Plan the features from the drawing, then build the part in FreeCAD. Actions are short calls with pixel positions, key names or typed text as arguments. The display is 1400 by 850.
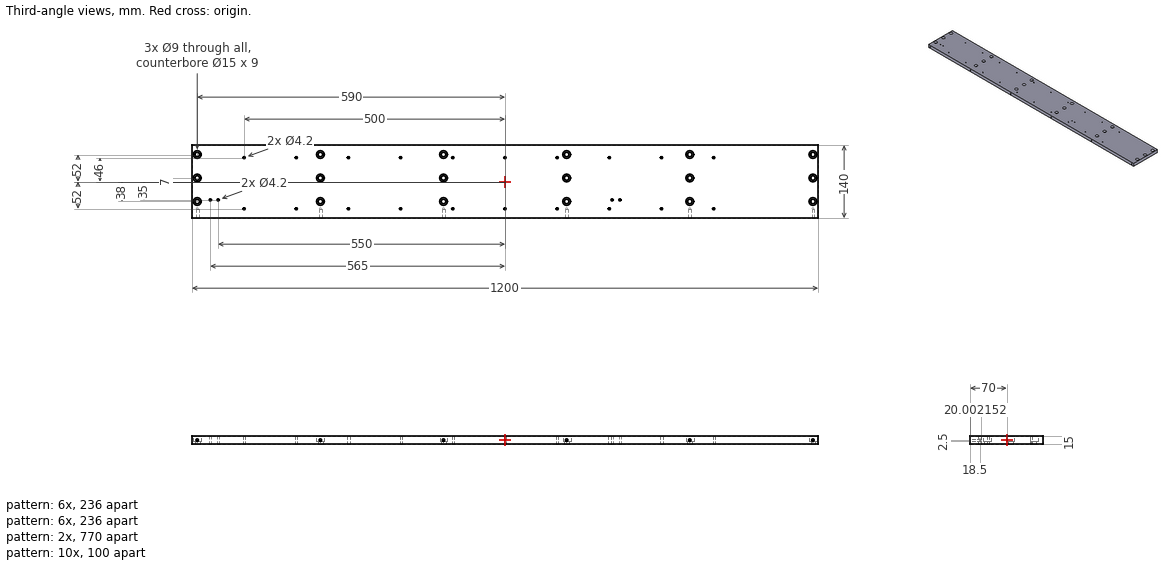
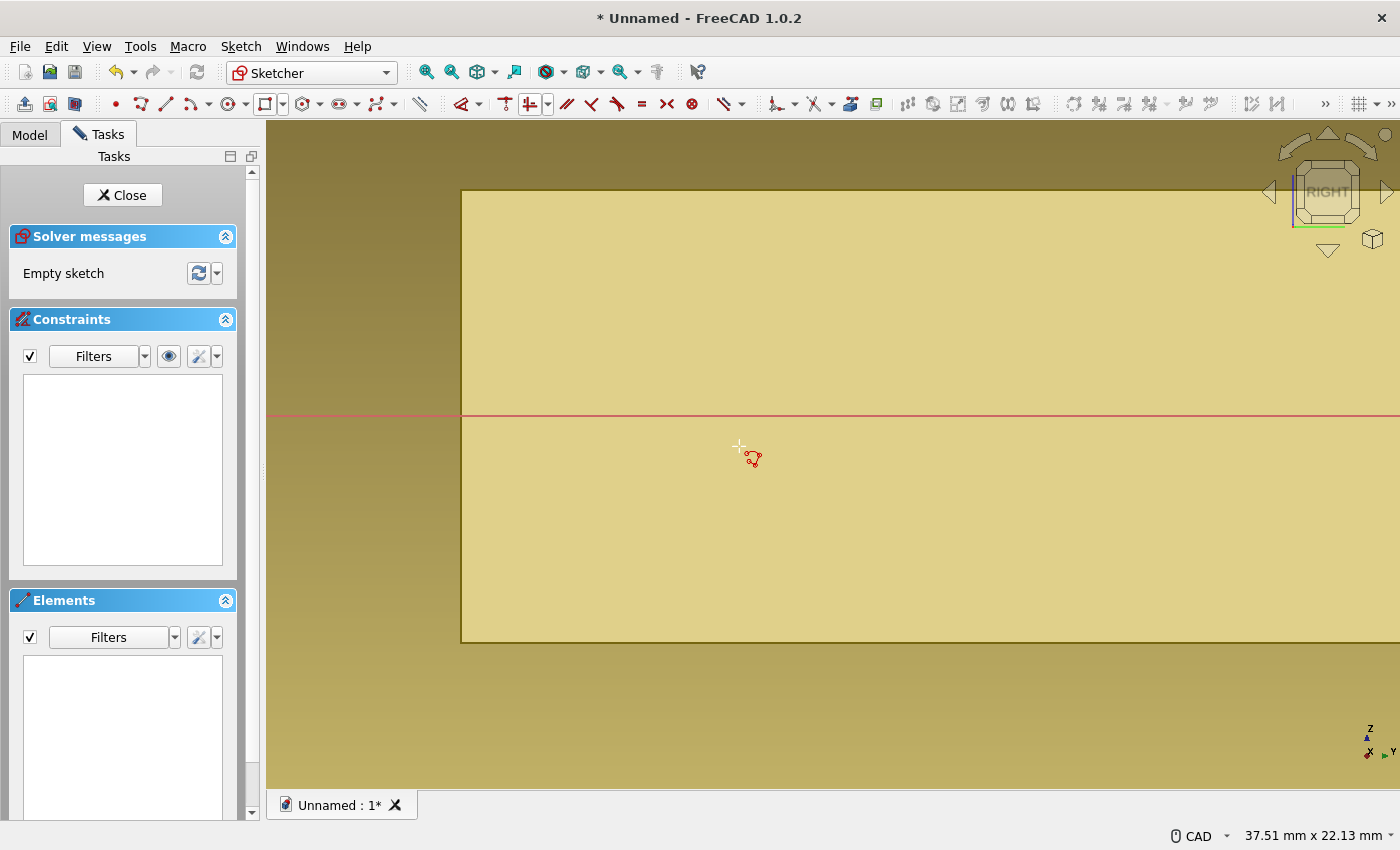
click(1066, 416)
click(461, 425)
click(461, 492)
click(1021, 492)
click(1066, 416)
key(Escape)
key(Escape)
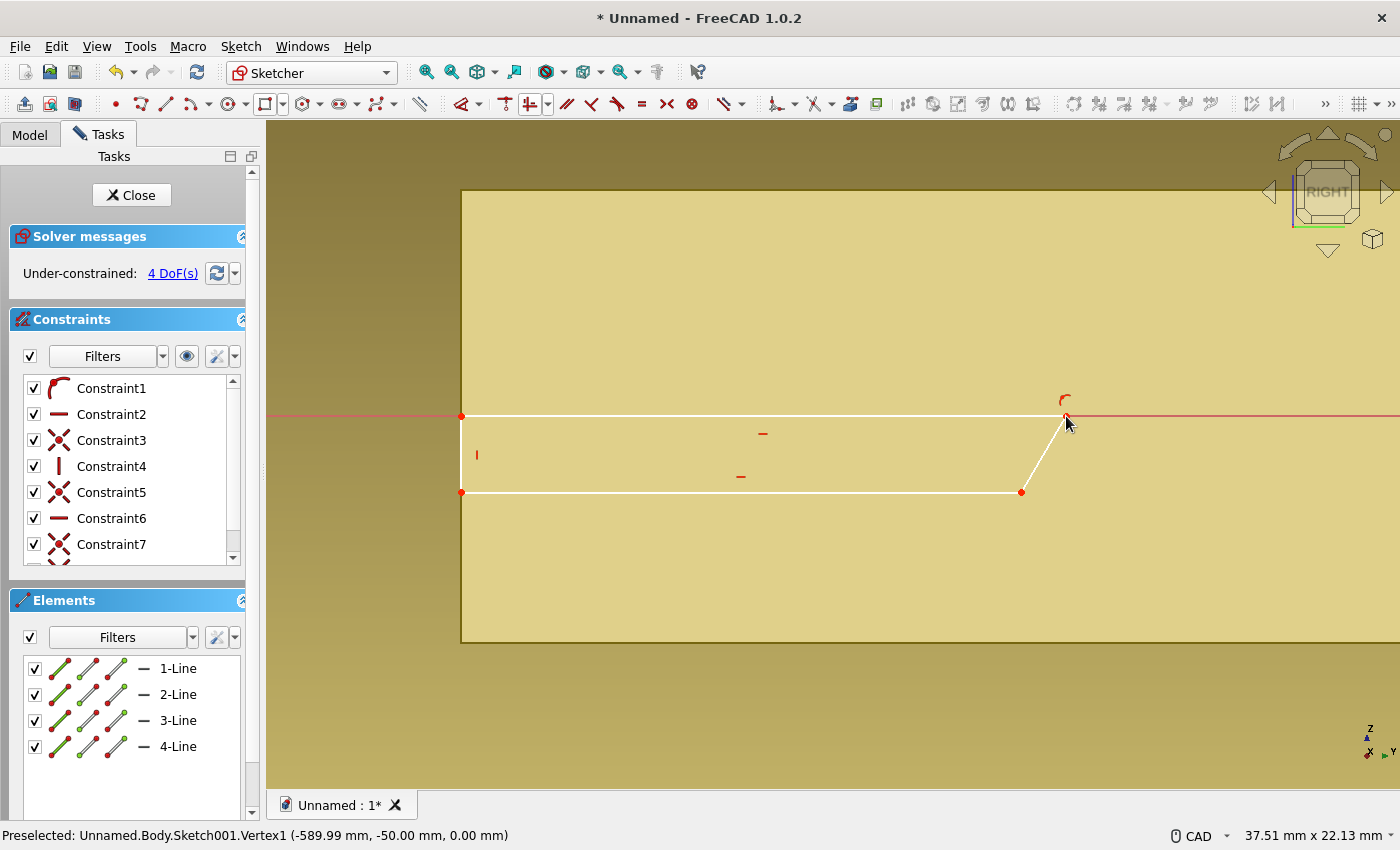
key(d)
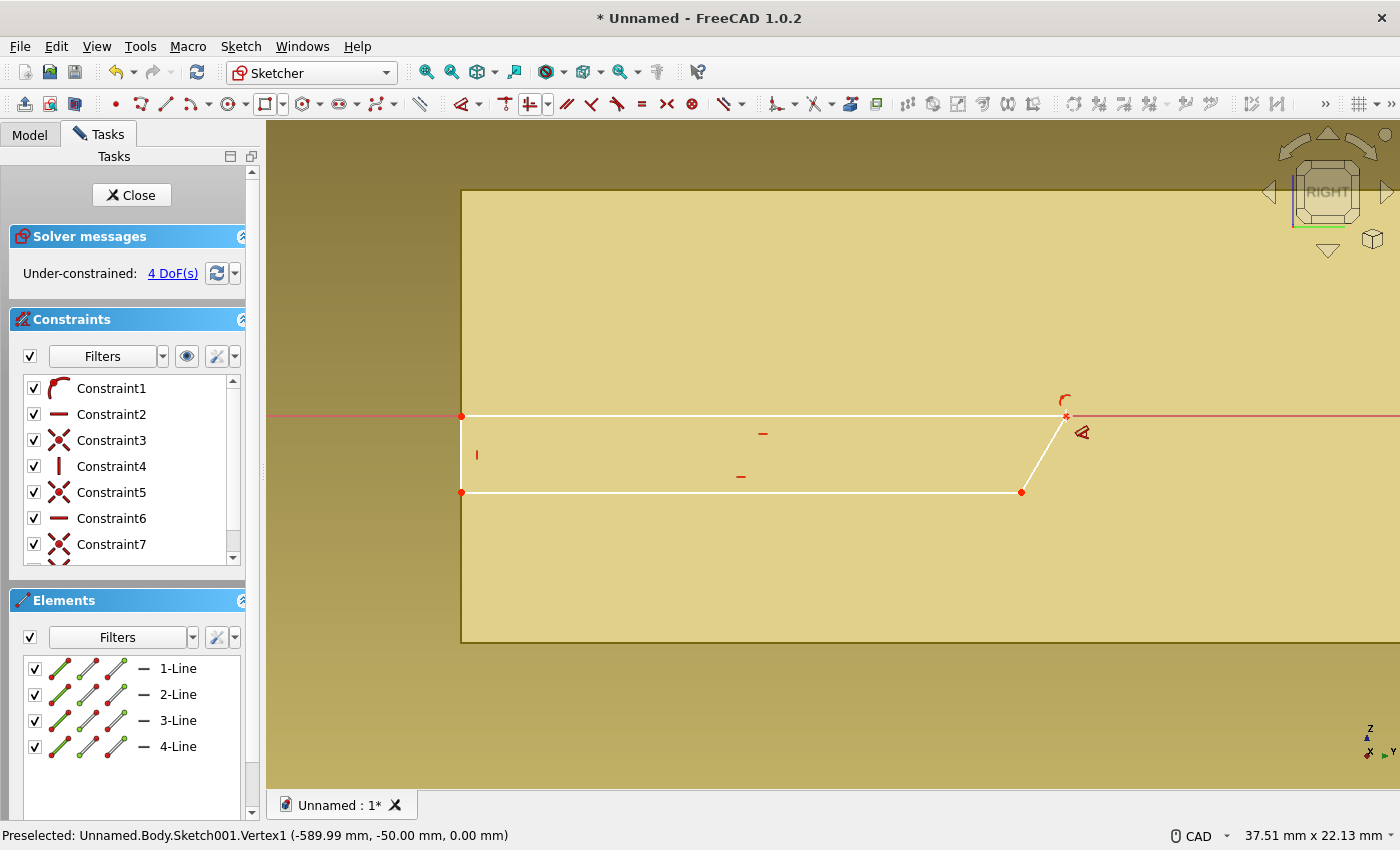
click(461, 439)
click(427, 455)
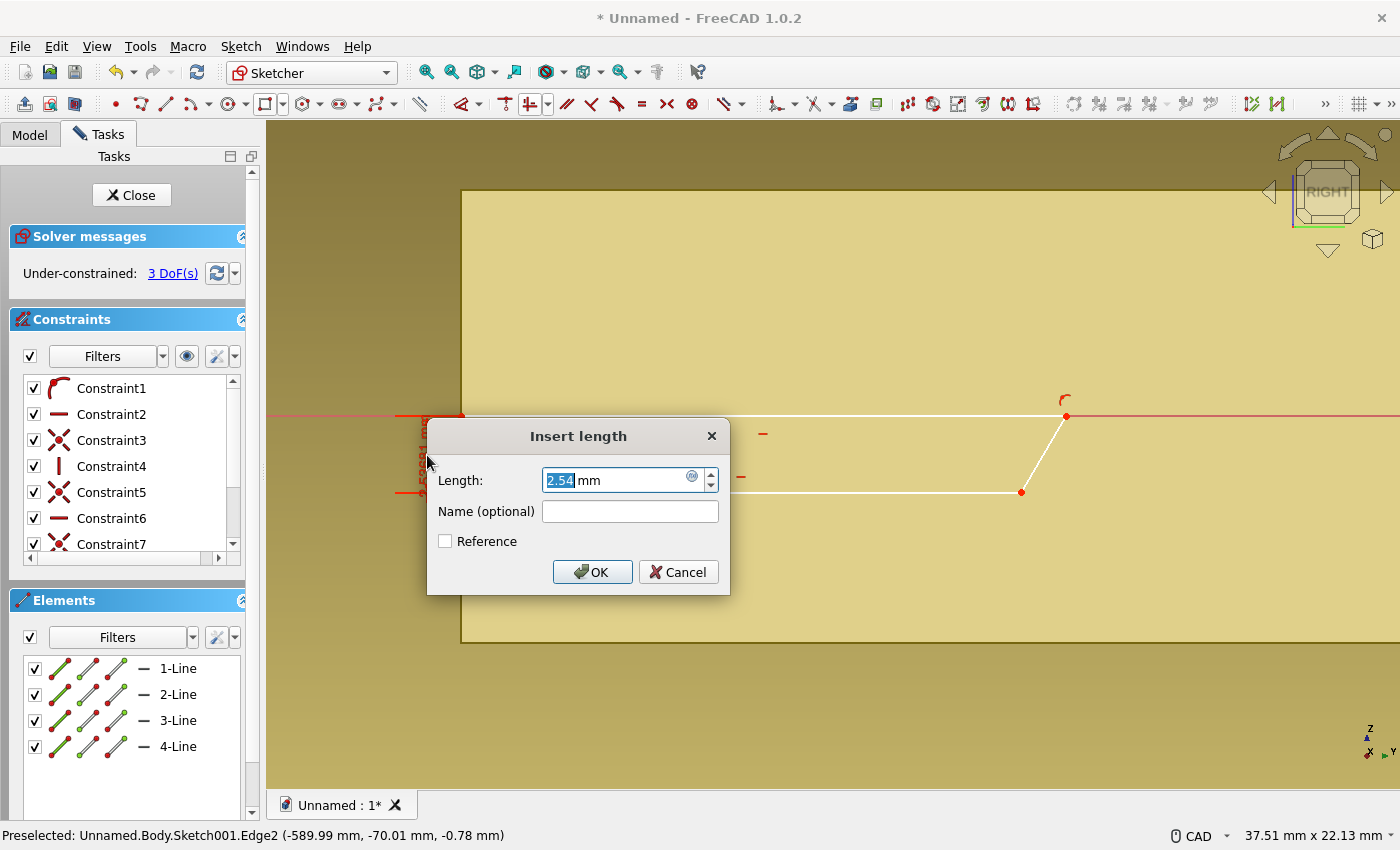
text(2.5)
key(Return)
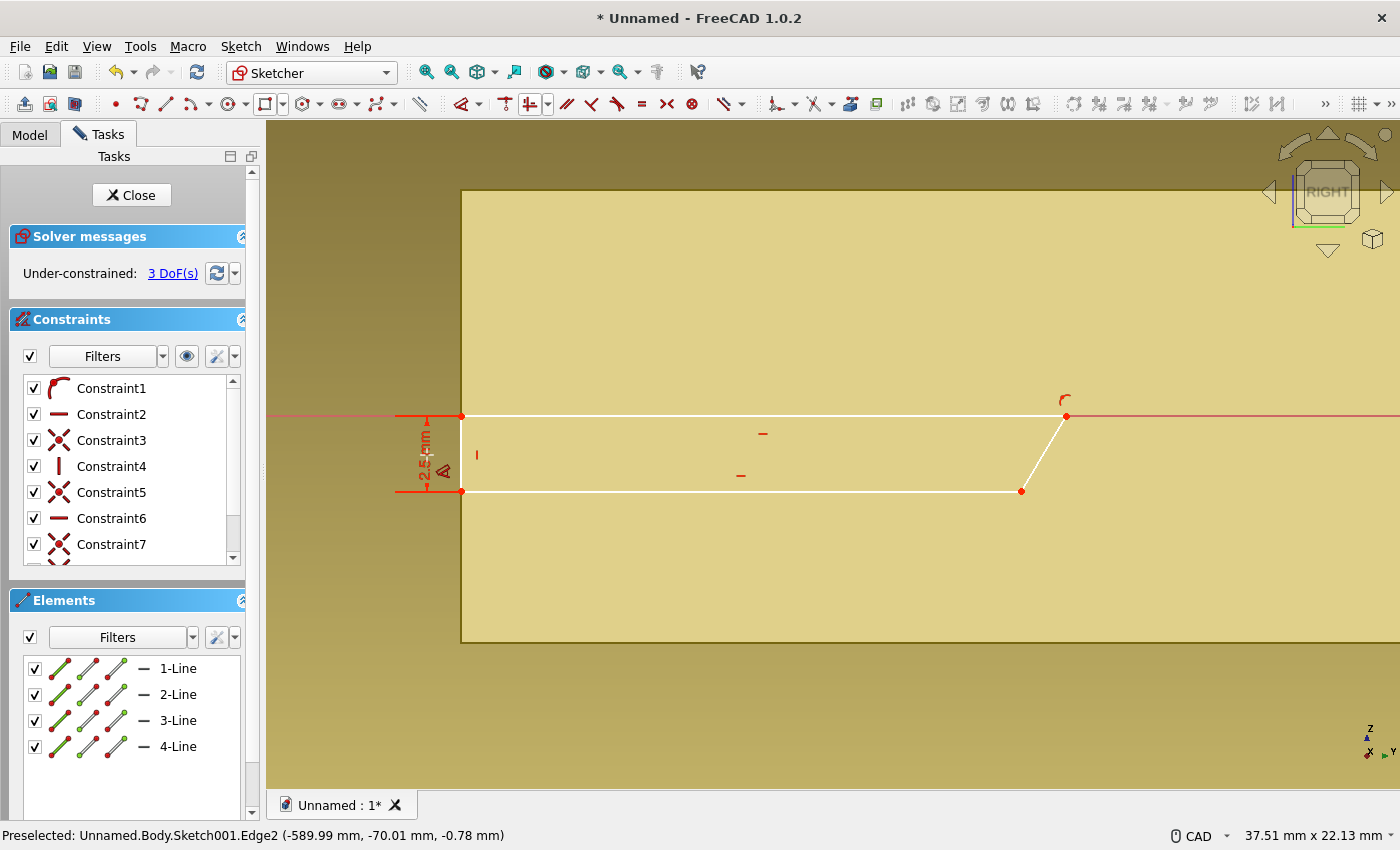
click(461, 416)
click(848, 382)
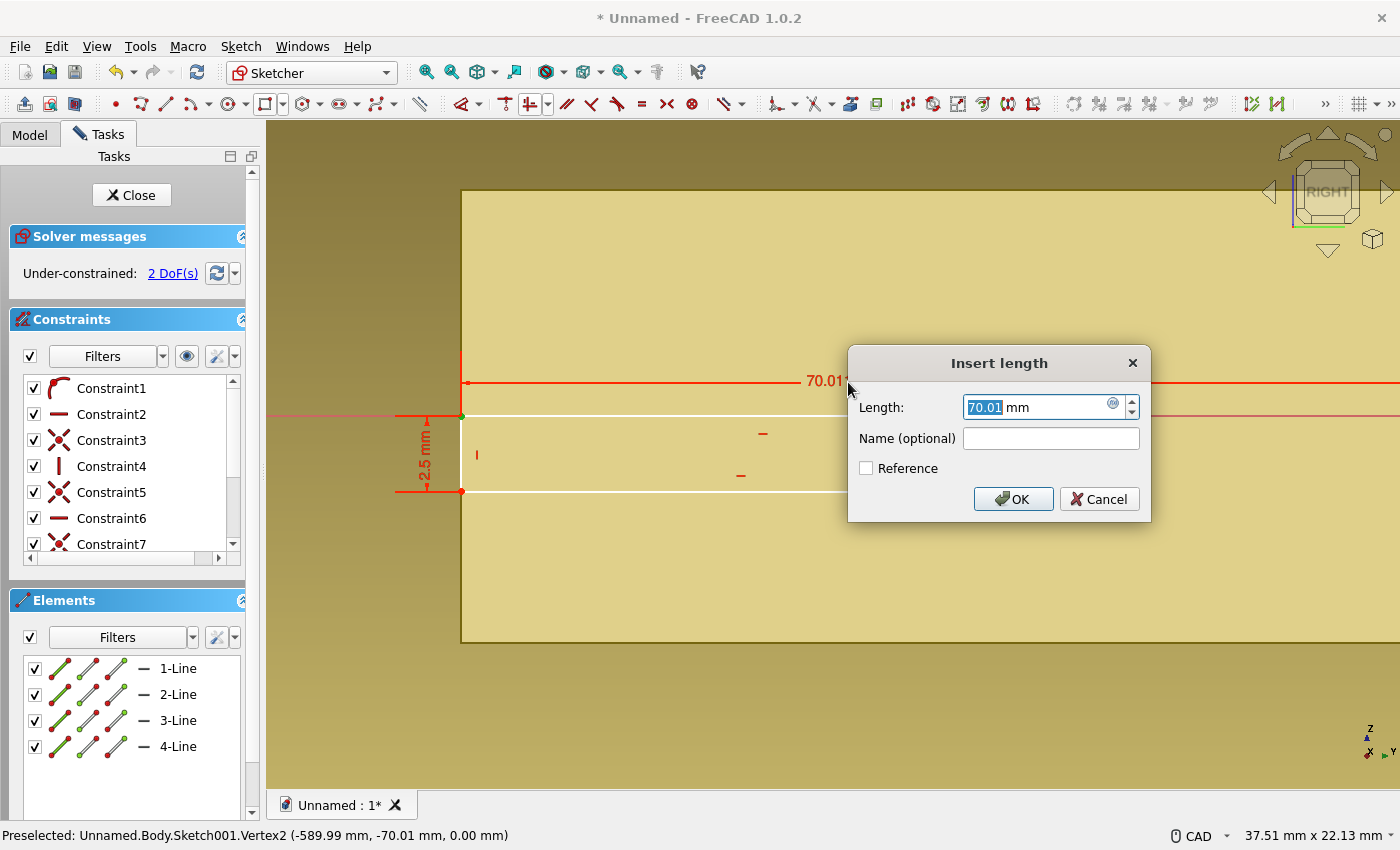
text(70)
key(Return)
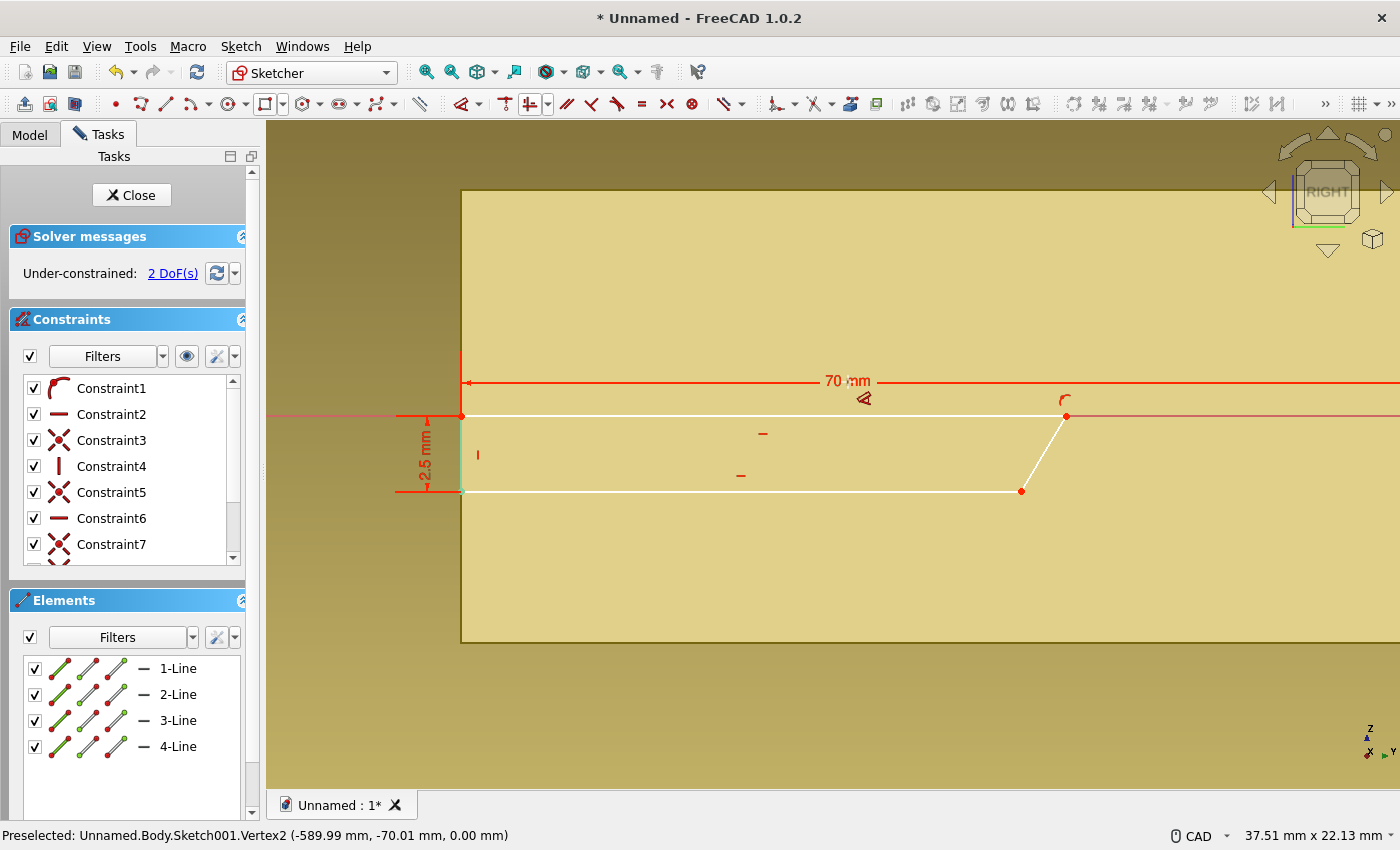
click(629, 492)
click(741, 526)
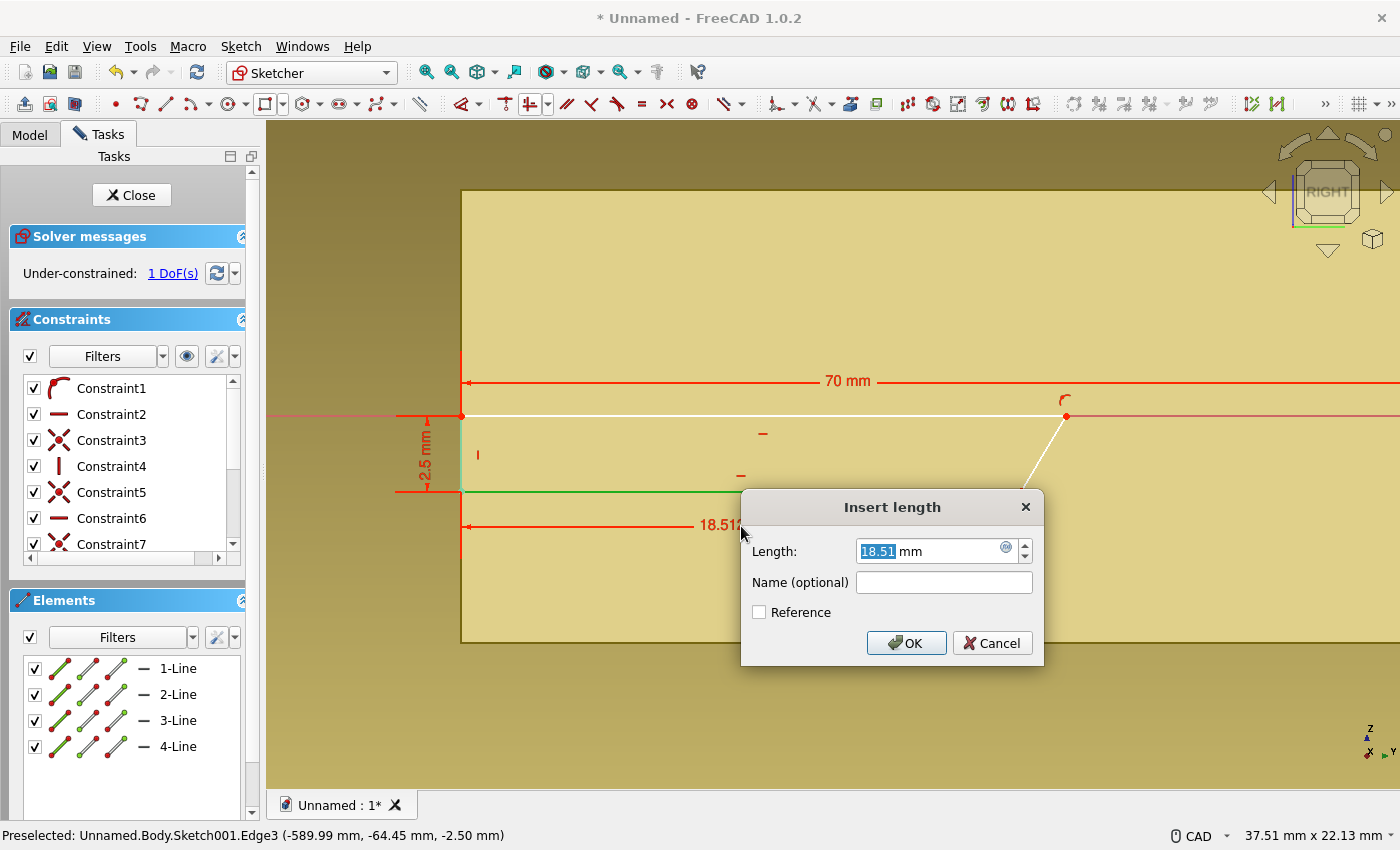
text(18.5)
key(Return)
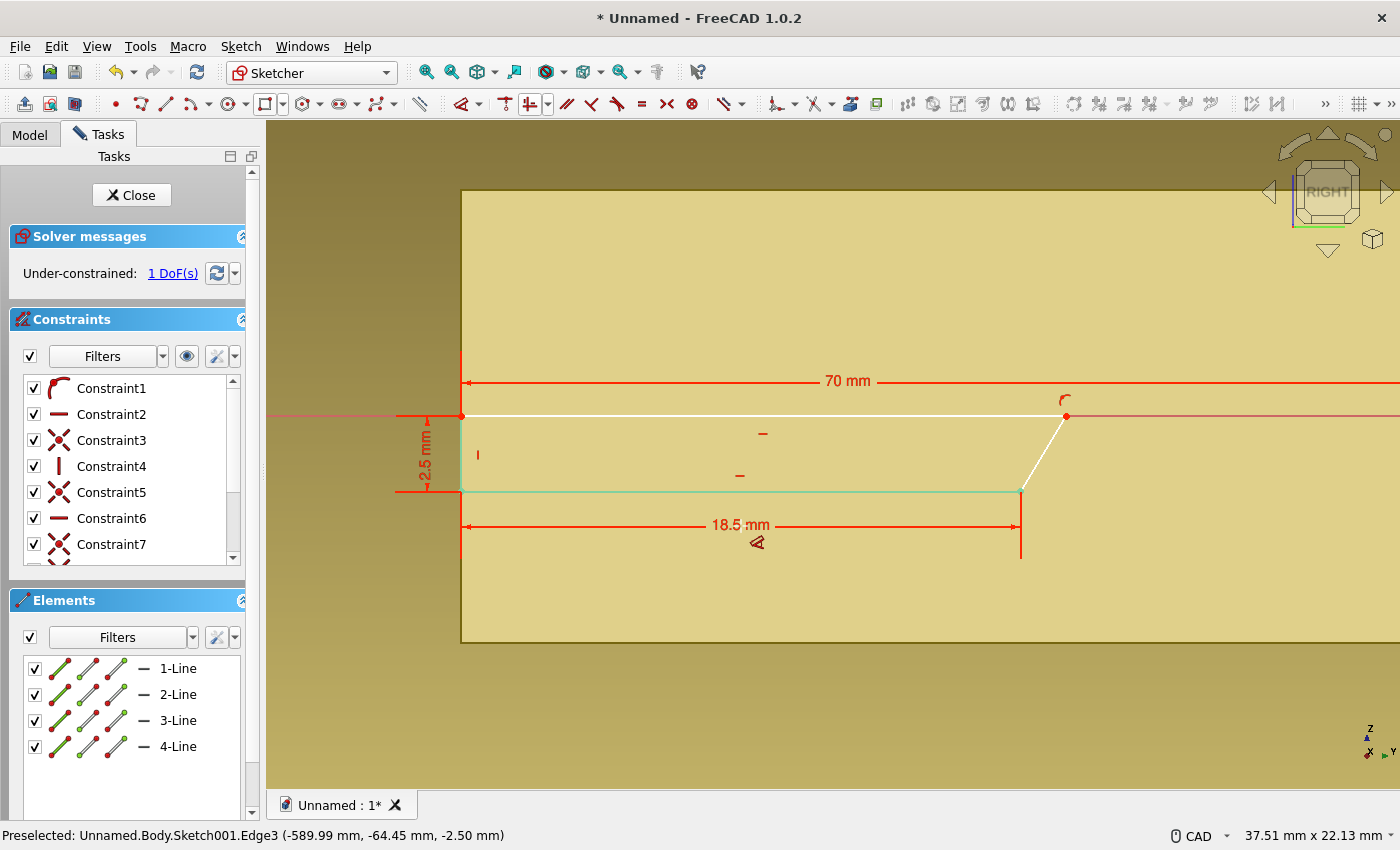
click(885, 416)
click(764, 382)